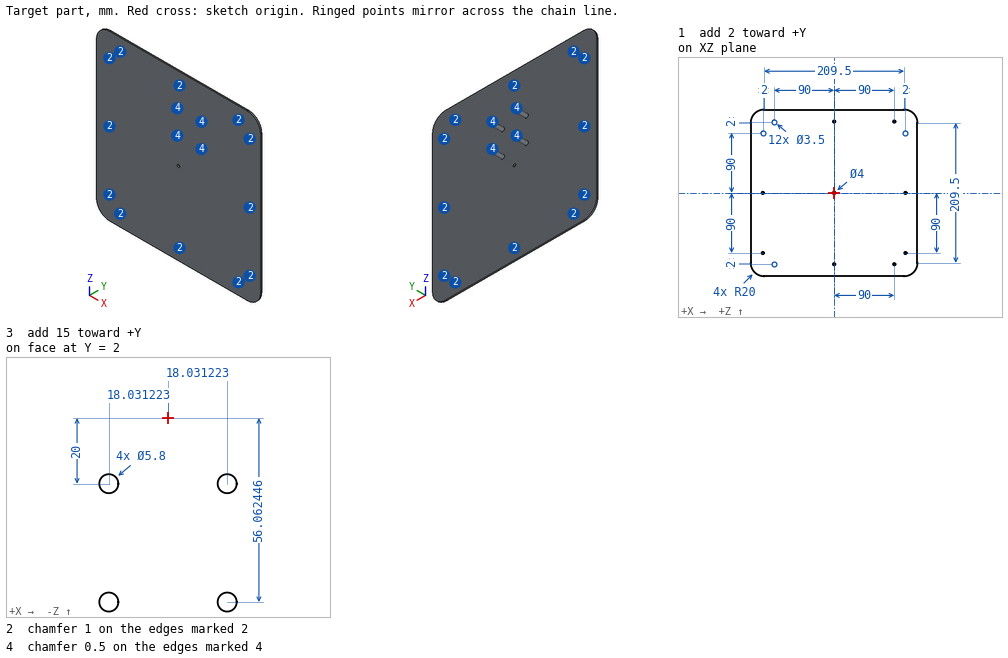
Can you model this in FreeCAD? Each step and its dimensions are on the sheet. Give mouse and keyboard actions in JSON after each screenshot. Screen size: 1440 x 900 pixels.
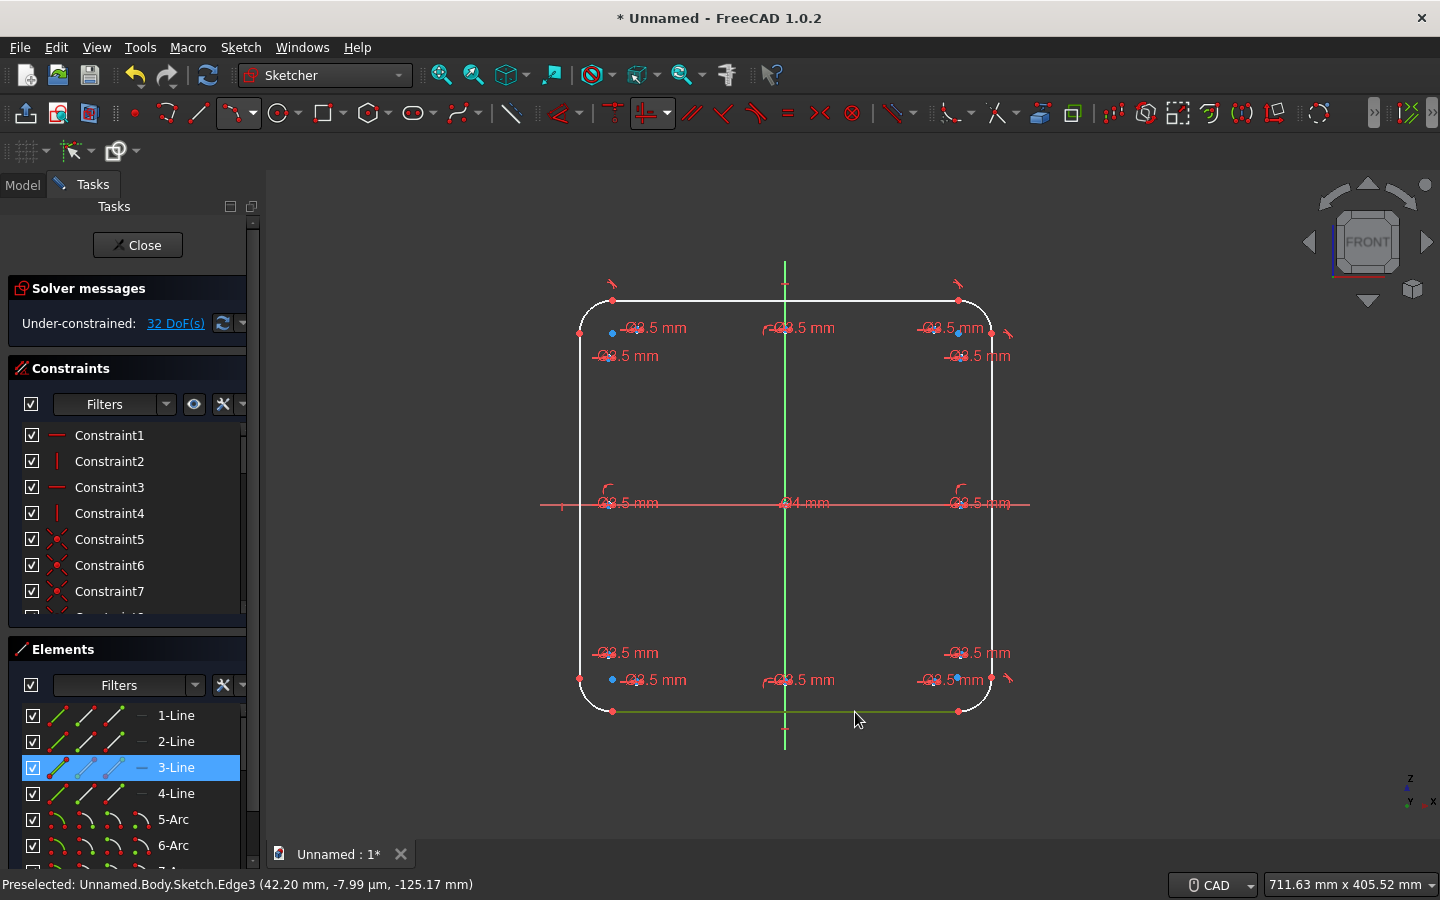
{"action": "left_click", "coordinate": [974, 708]}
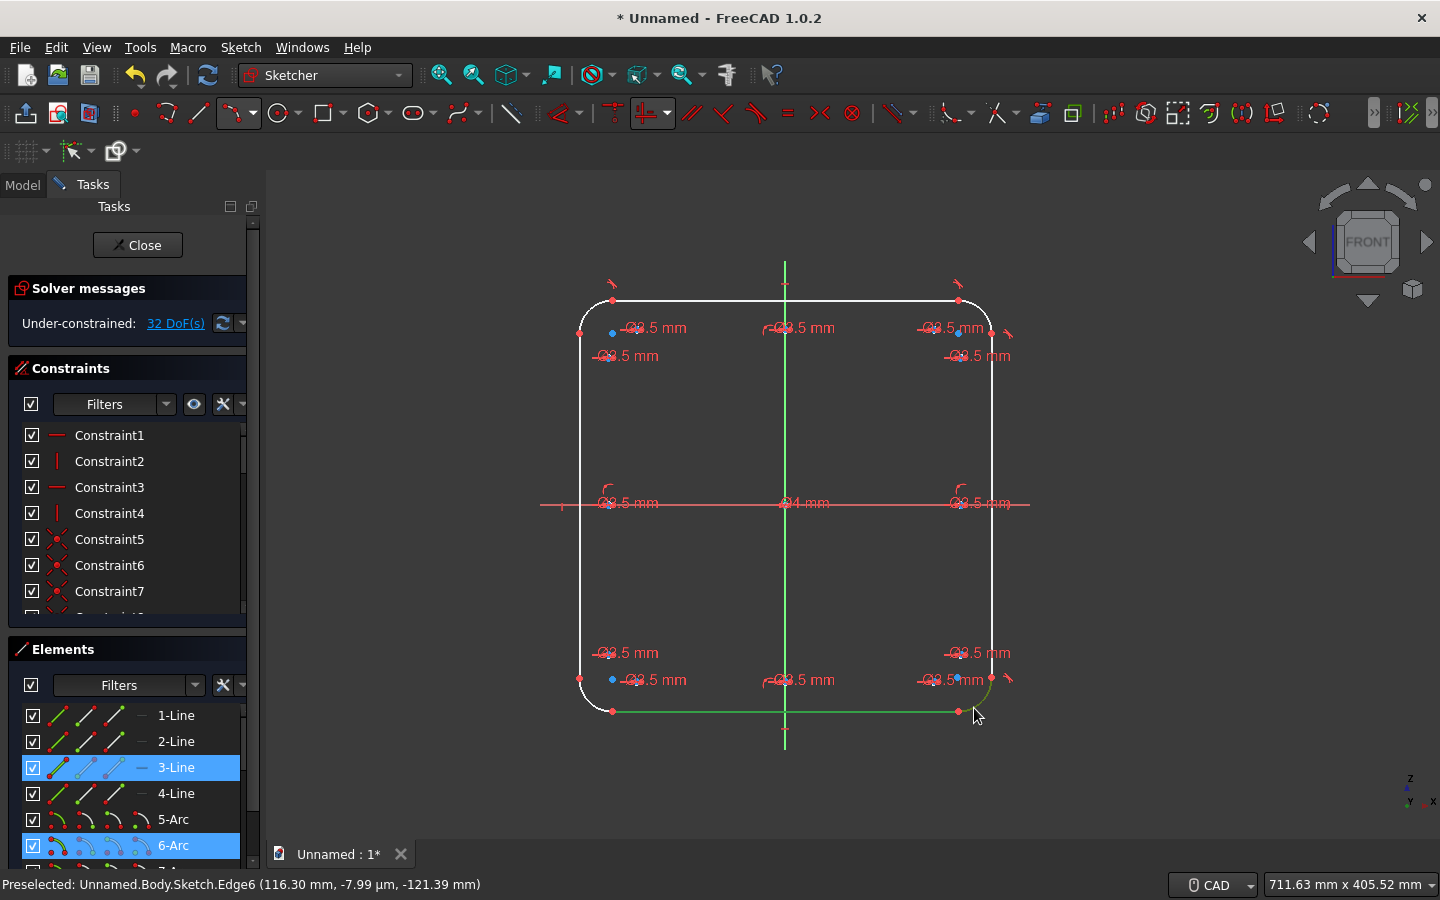
{"action": "key", "text": "t"}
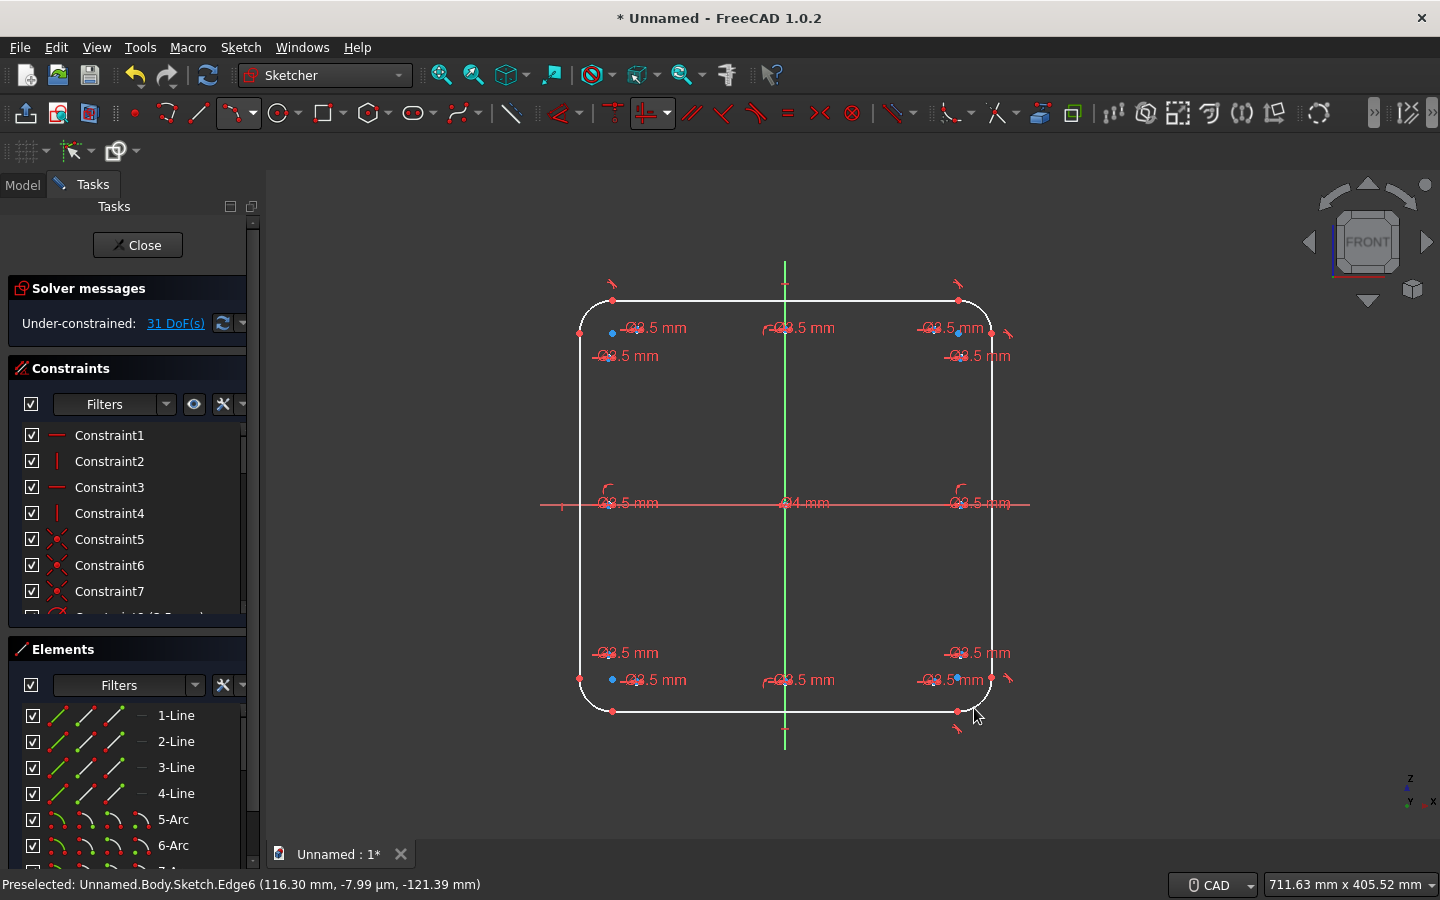
{"action": "left_click", "coordinate": [854, 712]}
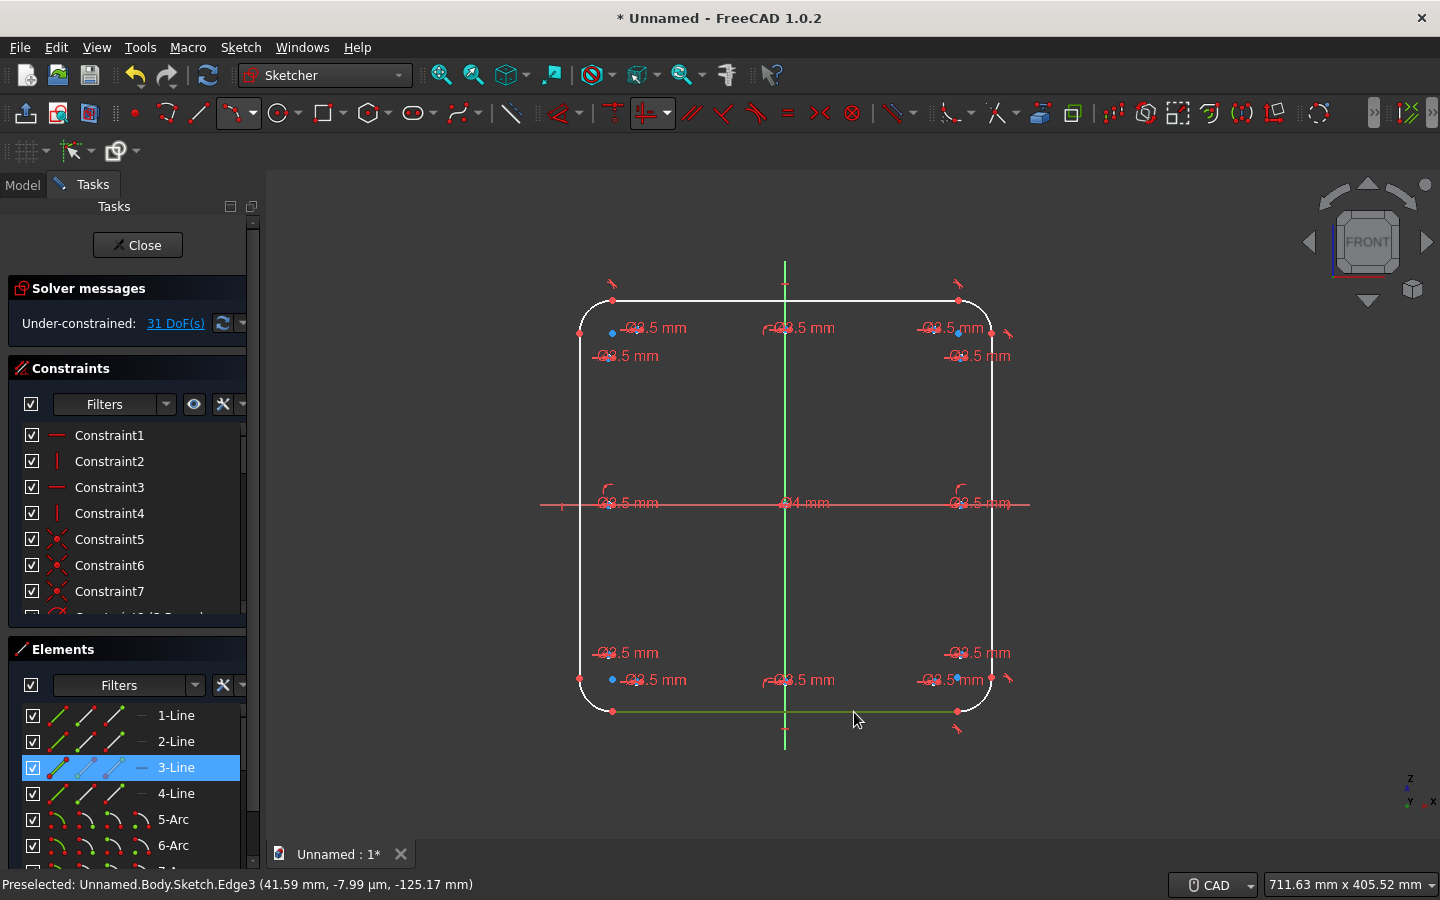
{"action": "left_click", "coordinate": [583, 694]}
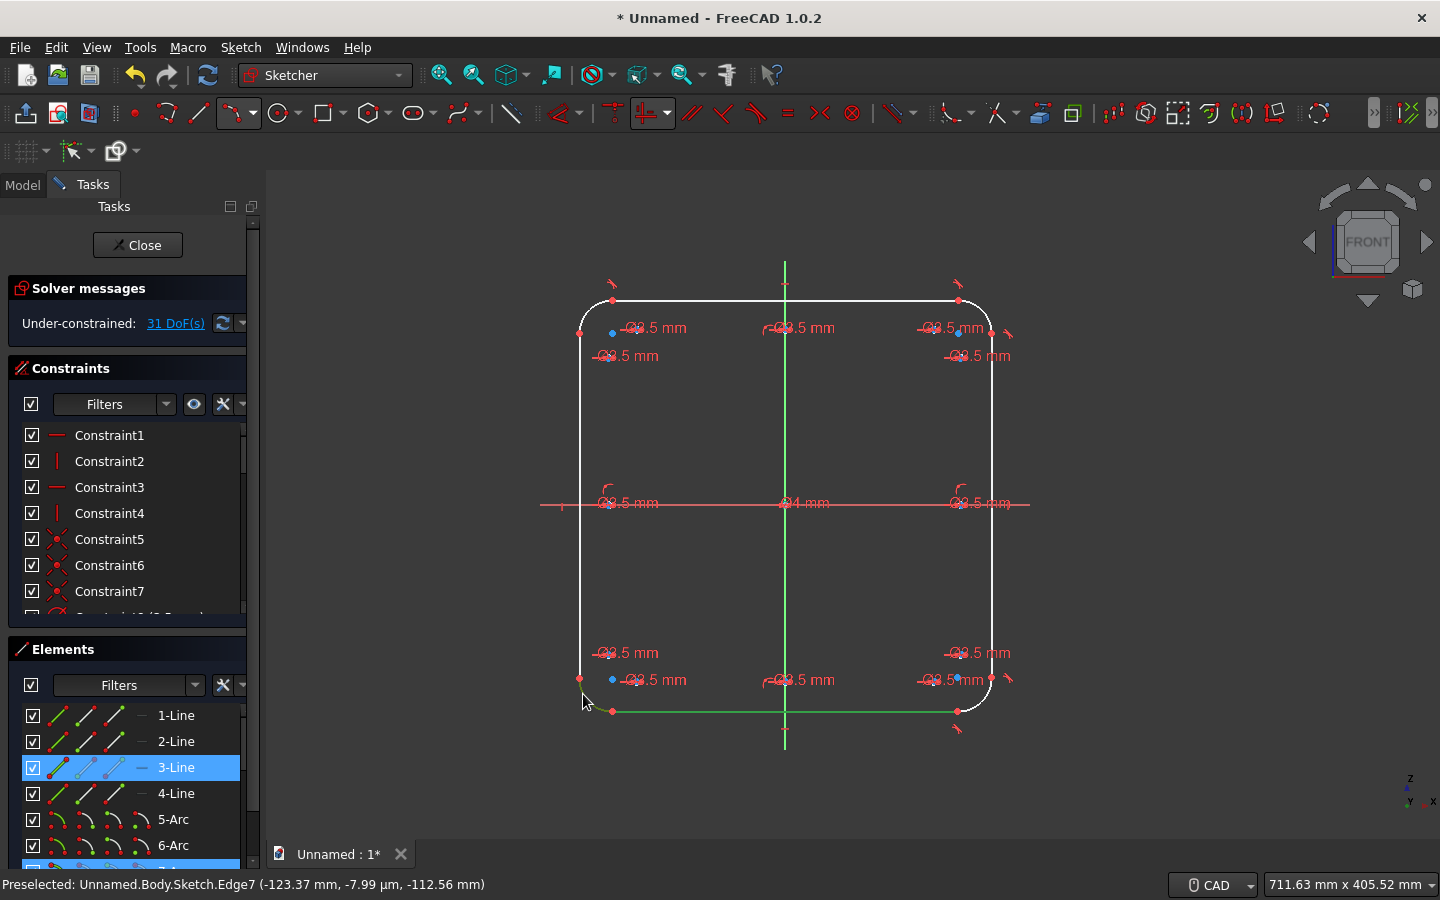
{"action": "key", "text": "t"}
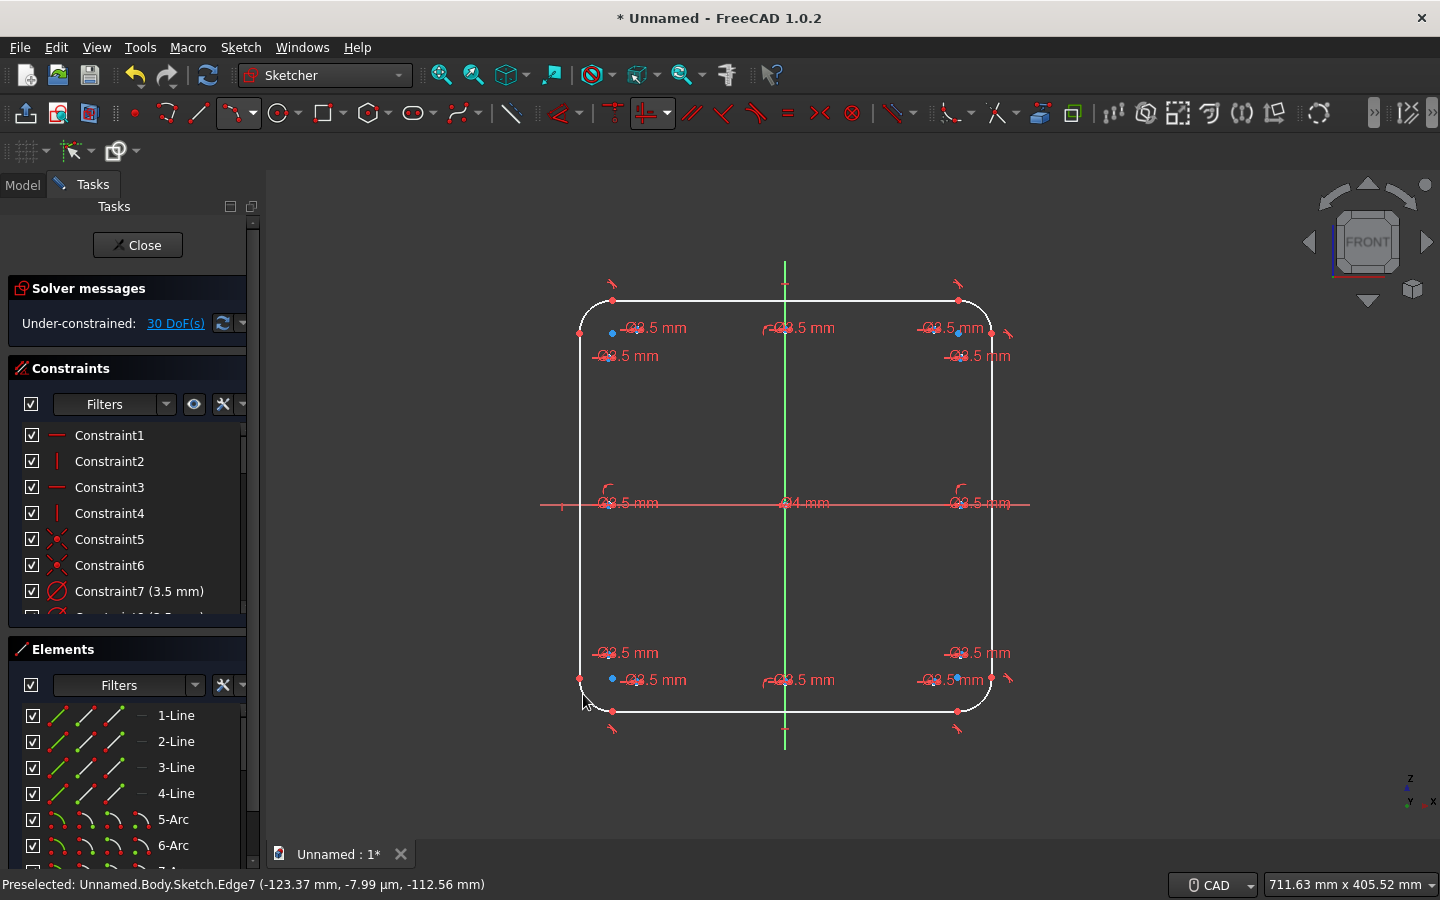
{"action": "left_click", "coordinate": [580, 575]}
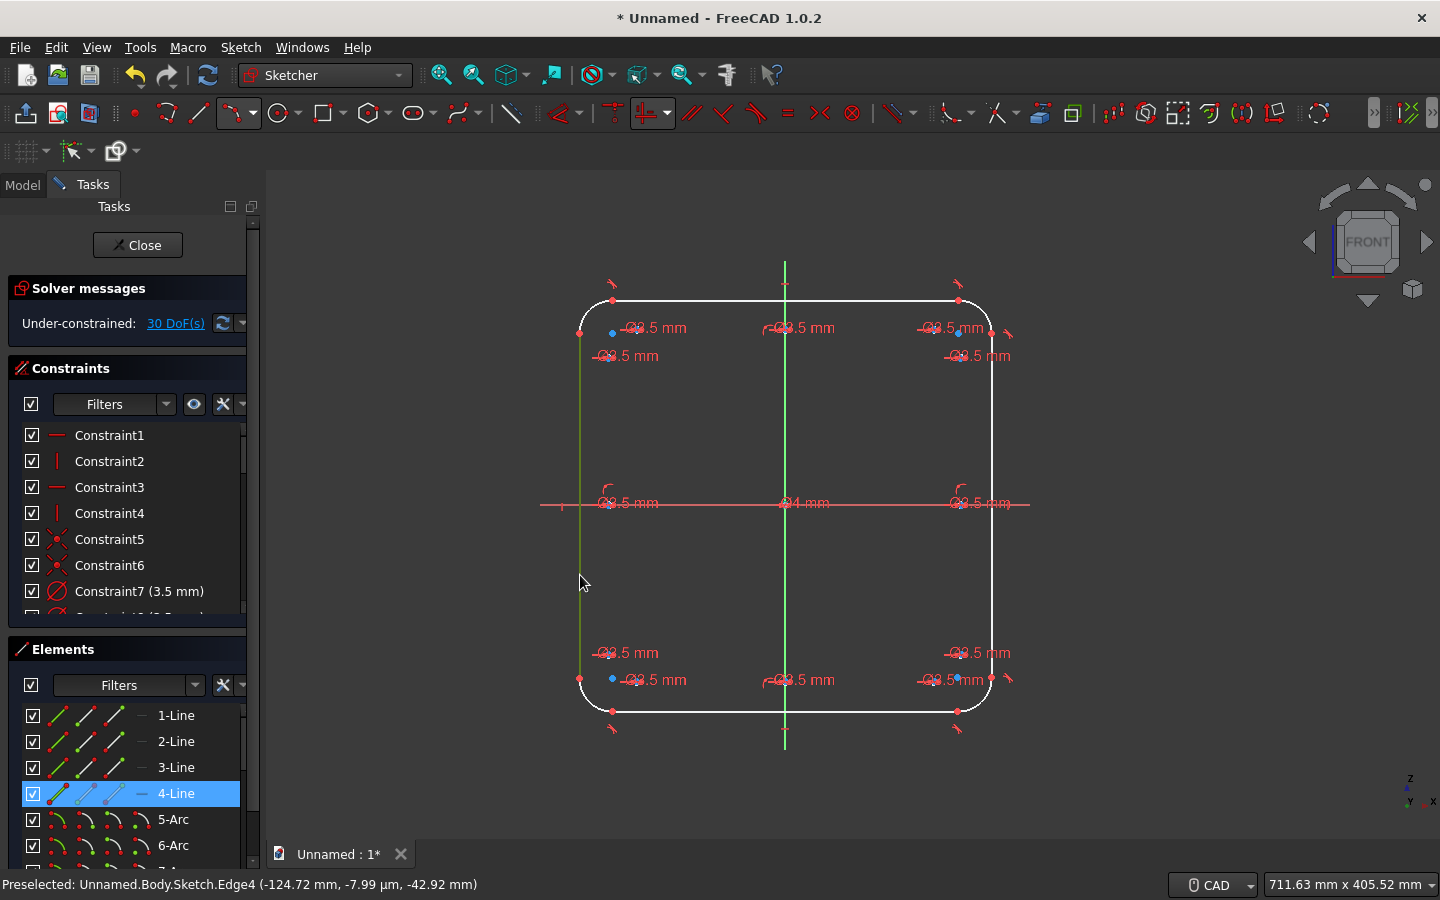
{"action": "left_click", "coordinate": [583, 694]}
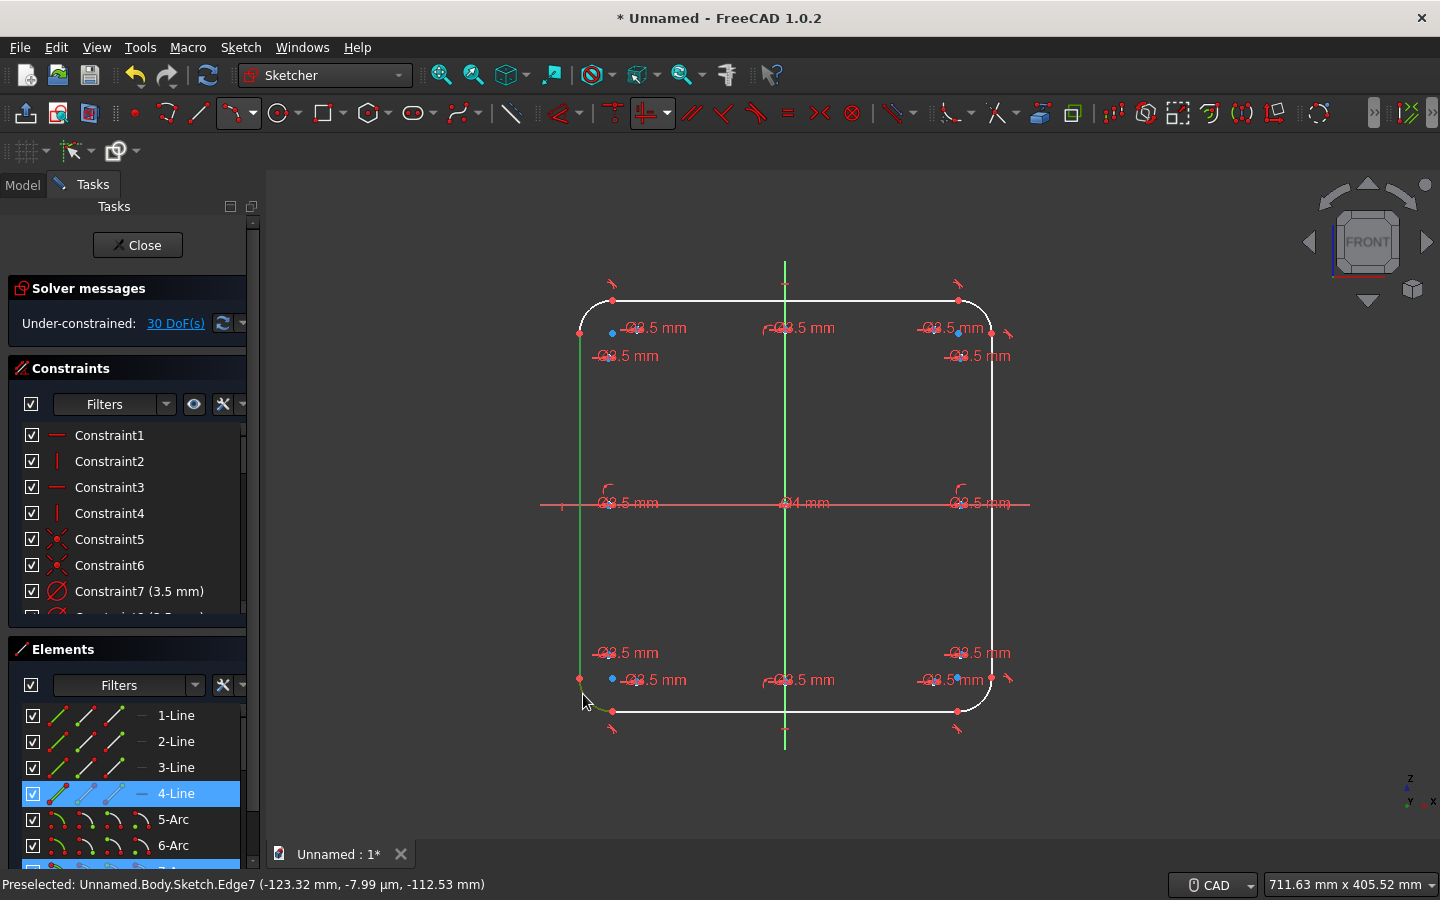
{"action": "key", "text": "t"}